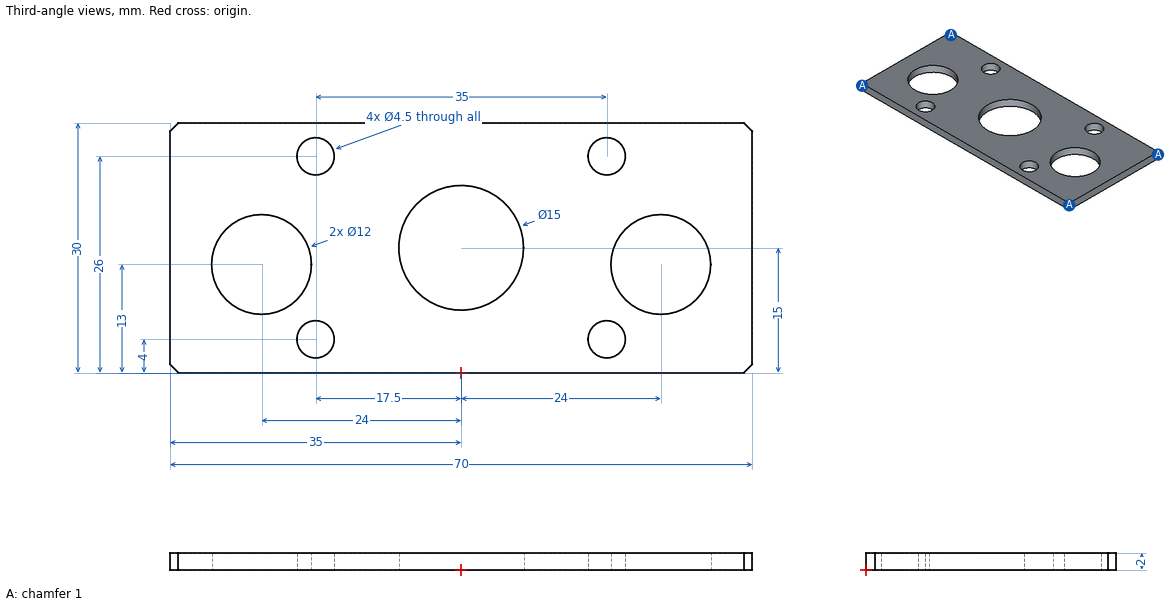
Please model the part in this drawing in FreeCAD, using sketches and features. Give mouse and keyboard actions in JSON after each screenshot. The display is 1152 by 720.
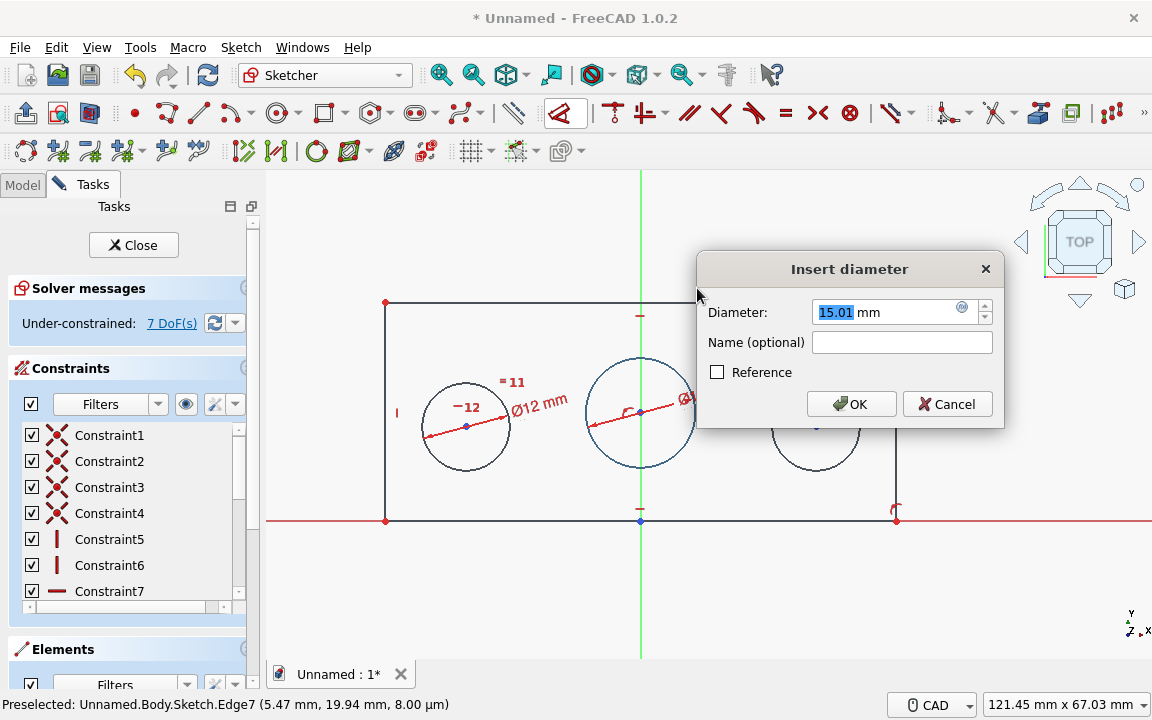
{"action": "type", "text": "15"}
{"action": "key", "text": "Return"}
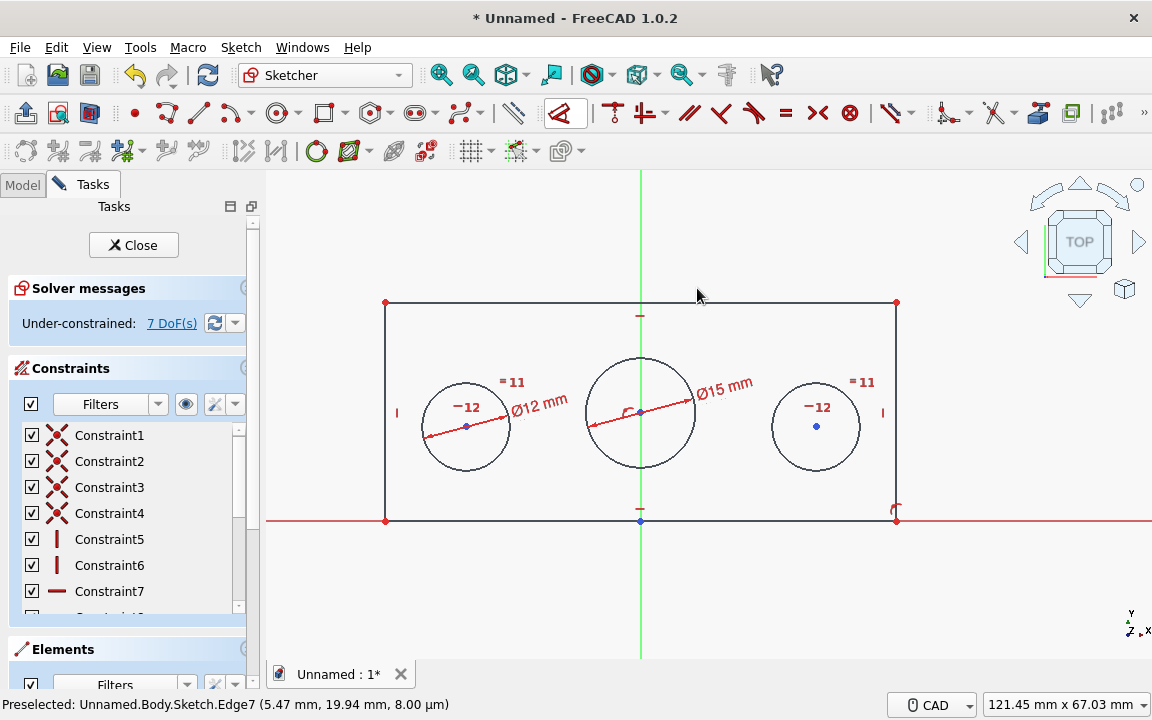
{"action": "left_click", "coordinate": [385, 368]}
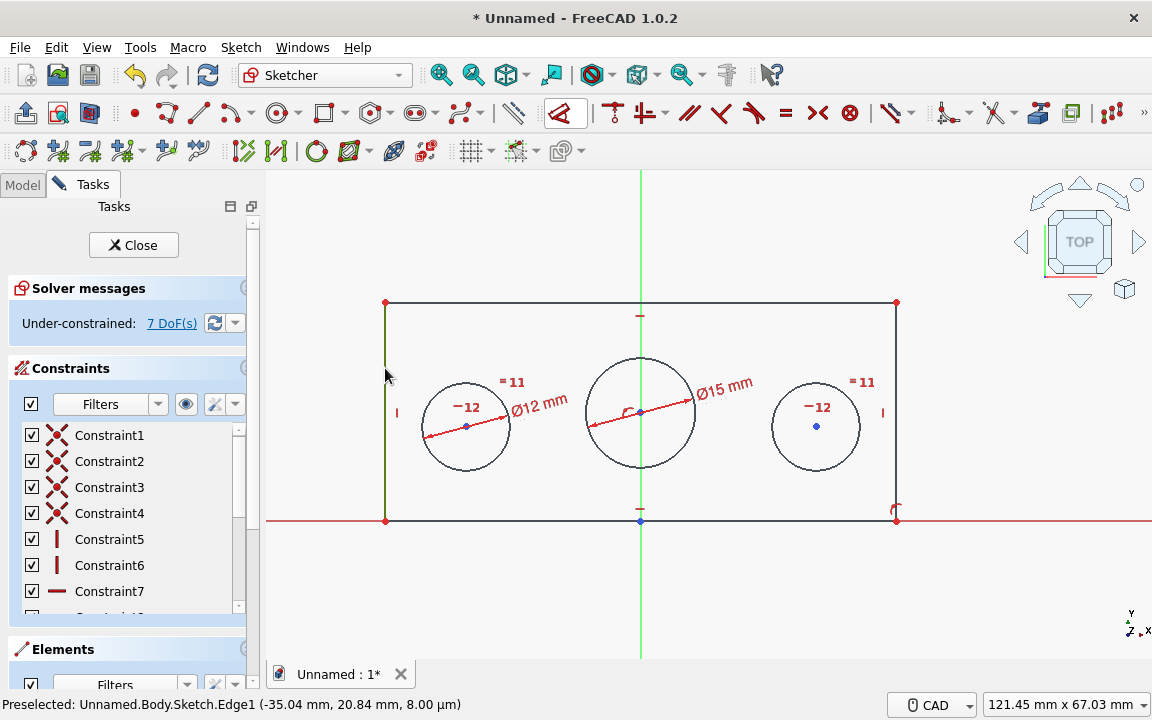
{"action": "key", "text": "i"}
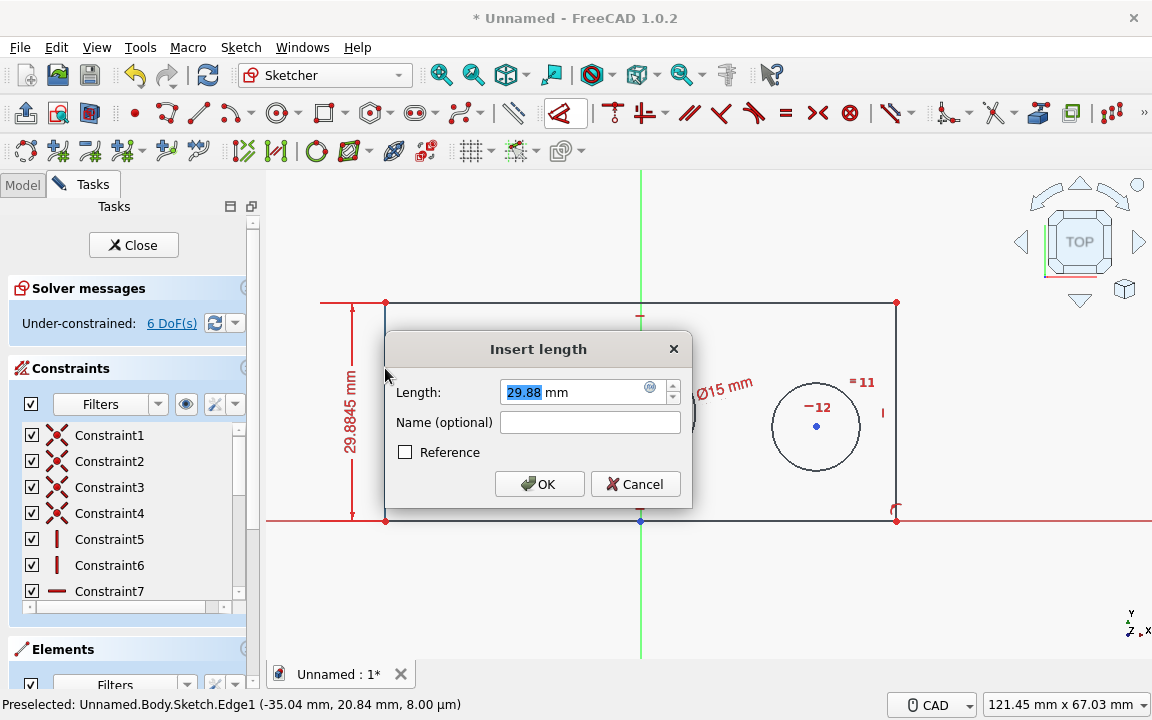
{"action": "type", "text": "30"}
{"action": "key", "text": "Return"}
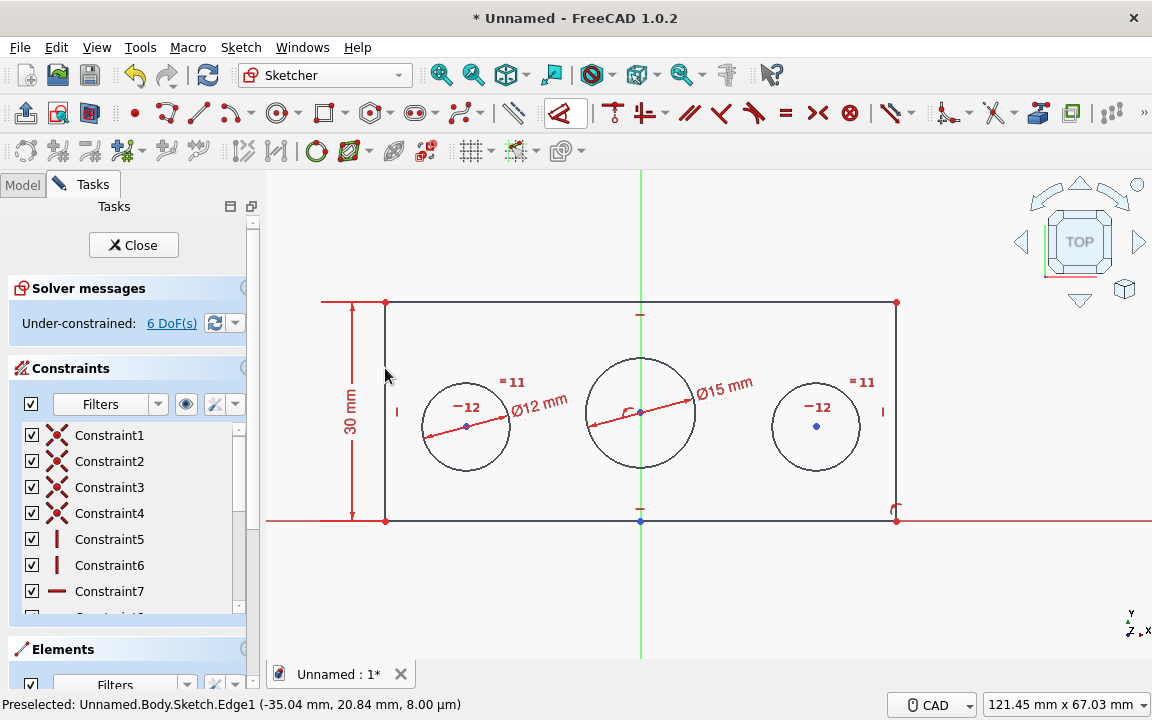
{"action": "left_click", "coordinate": [538, 521]}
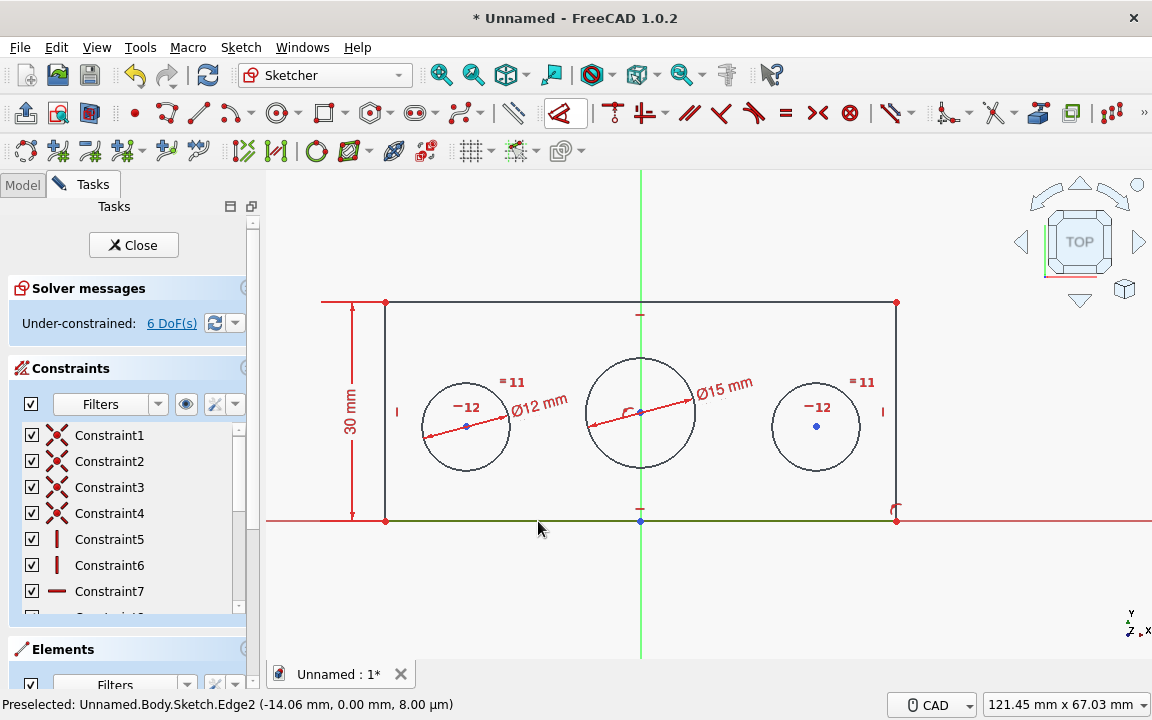
{"action": "key", "text": "l"}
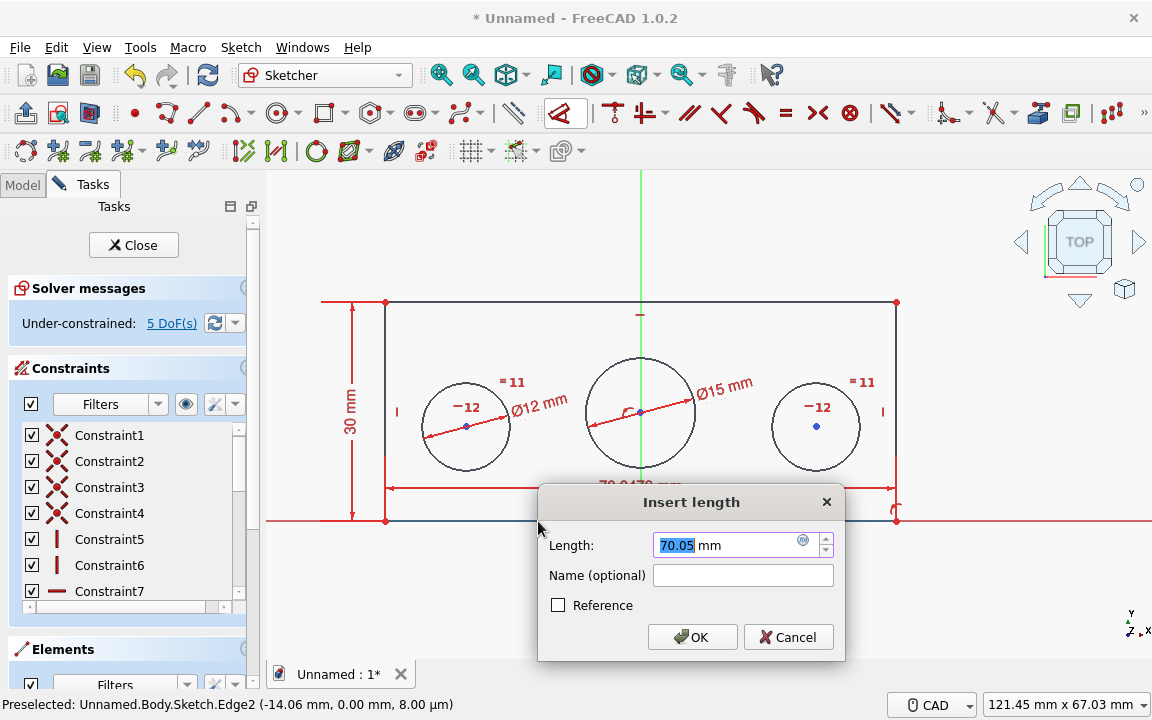
{"action": "type", "text": "70"}
{"action": "key", "text": "Return"}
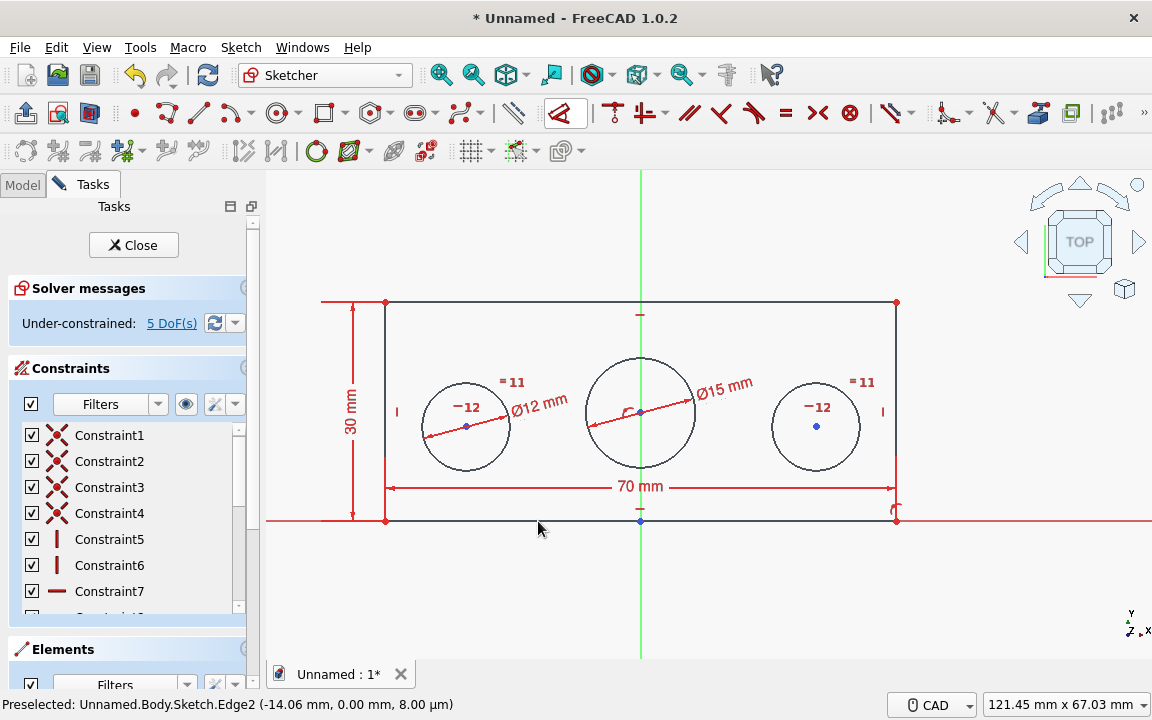
{"action": "left_click", "coordinate": [466, 427]}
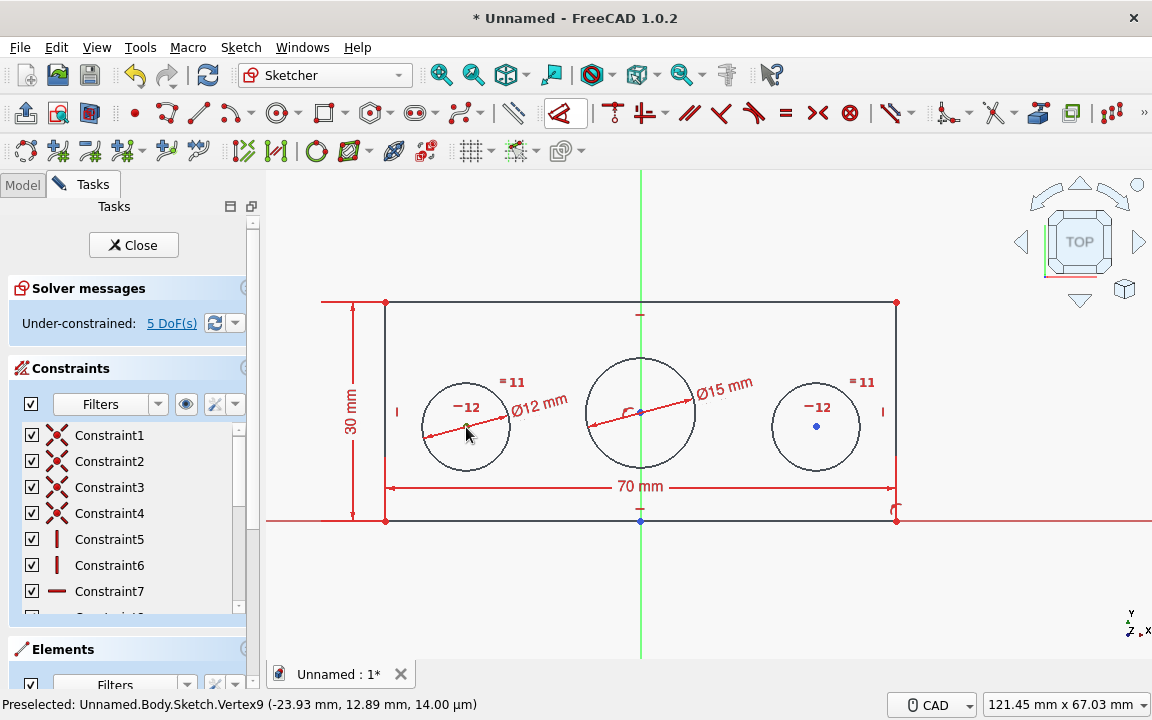
{"action": "key", "text": "l"}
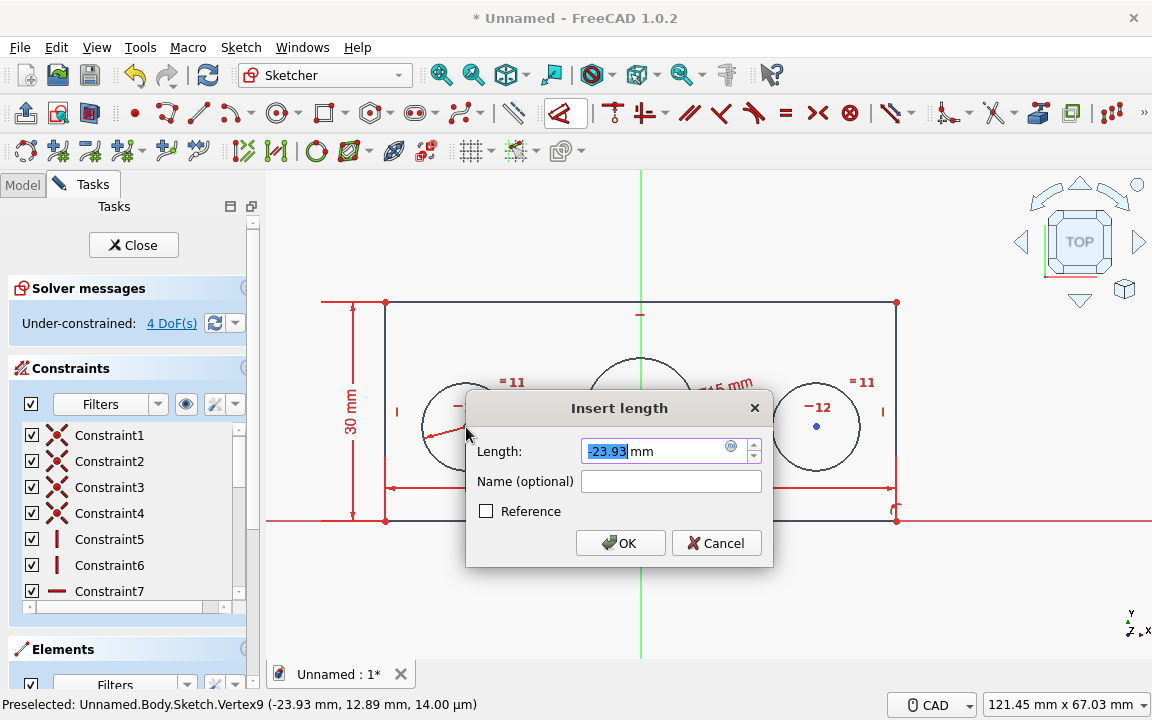
{"action": "type", "text": "-24"}
{"action": "key", "text": "Return"}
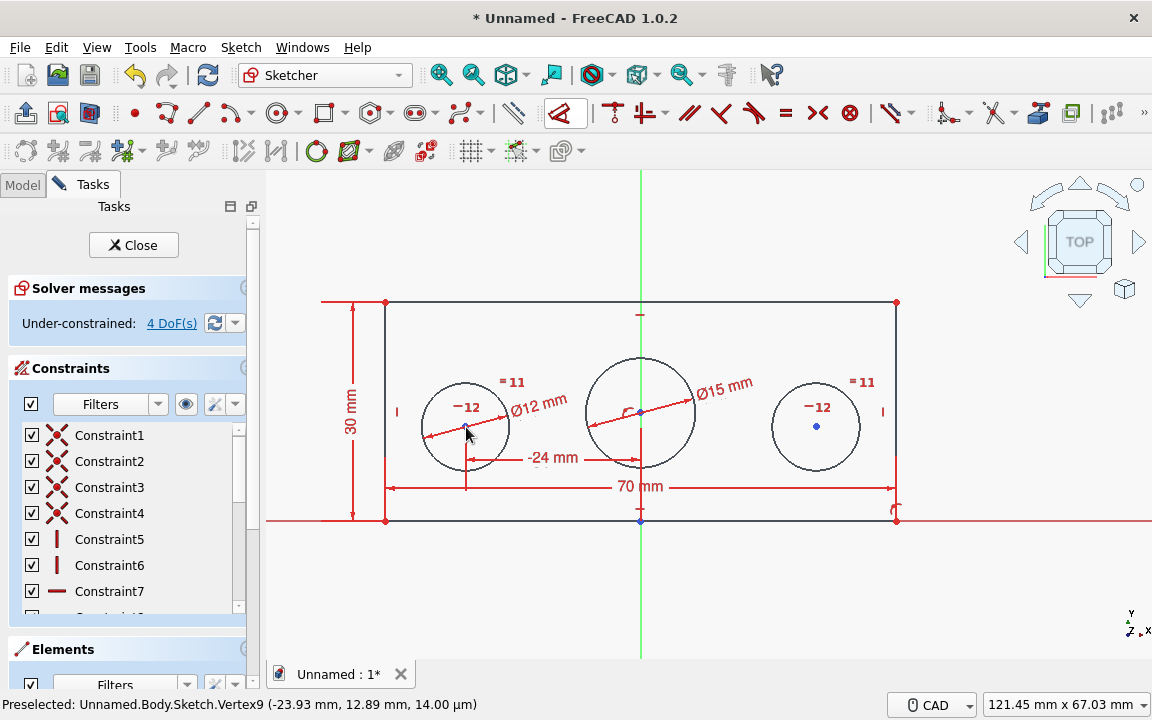
{"action": "left_click", "coordinate": [466, 427]}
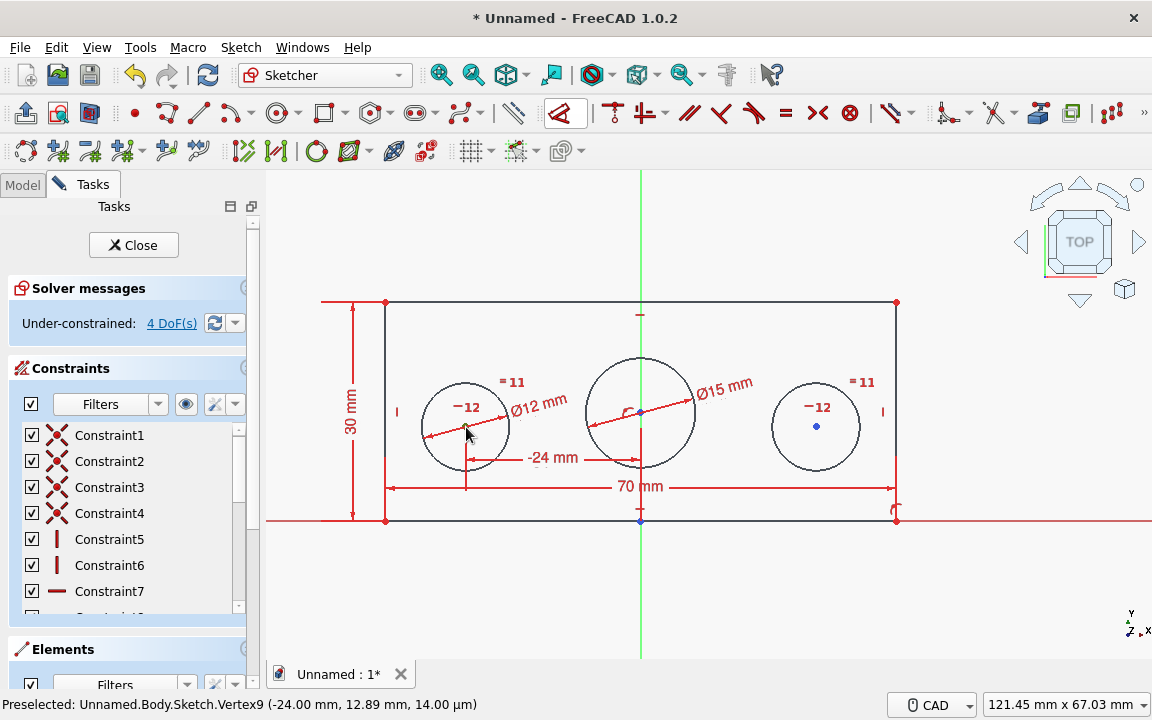
{"action": "key", "text": "i"}